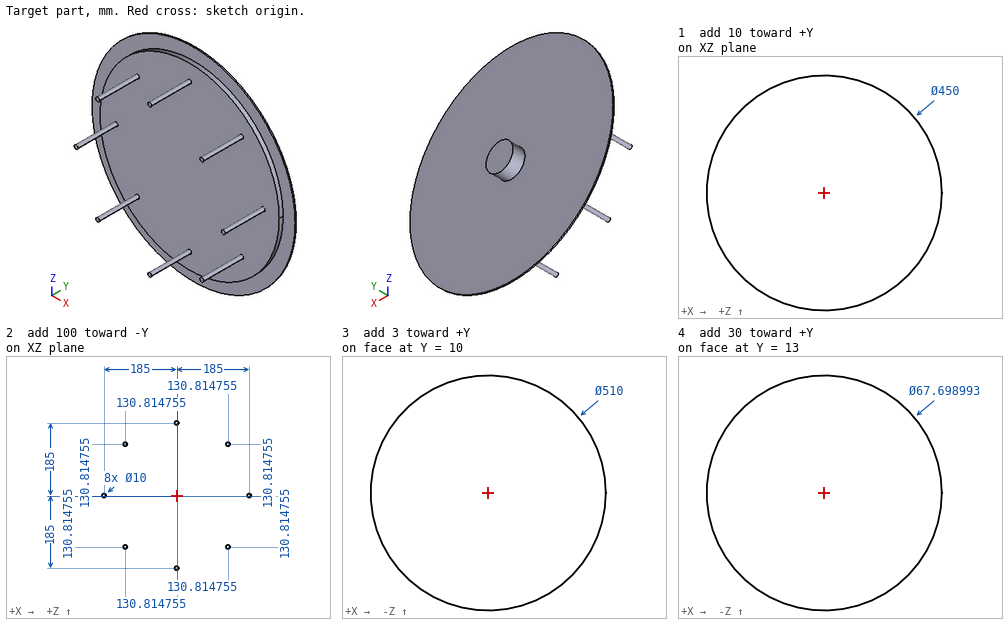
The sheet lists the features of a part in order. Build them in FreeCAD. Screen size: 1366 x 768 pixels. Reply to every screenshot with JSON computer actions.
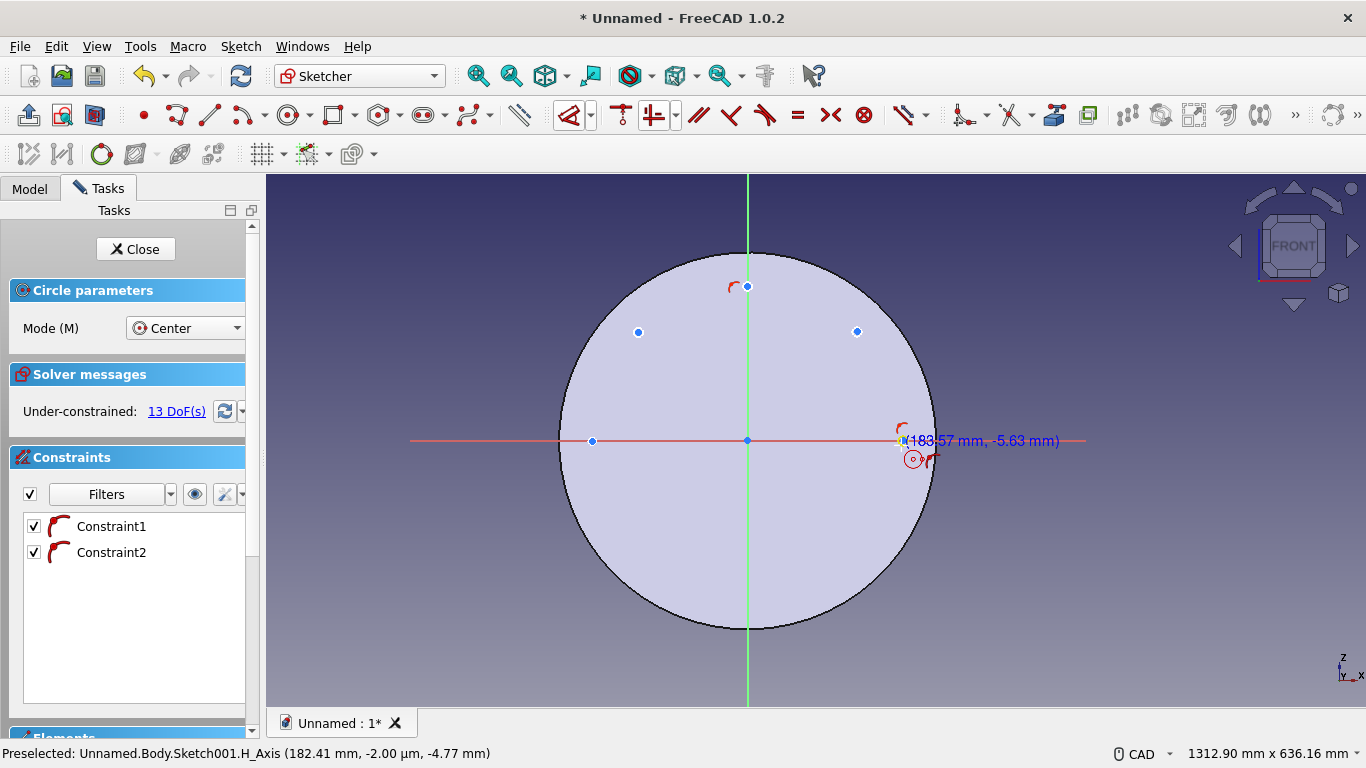
{"action": "scroll", "coordinate": [857, 551], "scroll_direction": "up", "scroll_amount": 9}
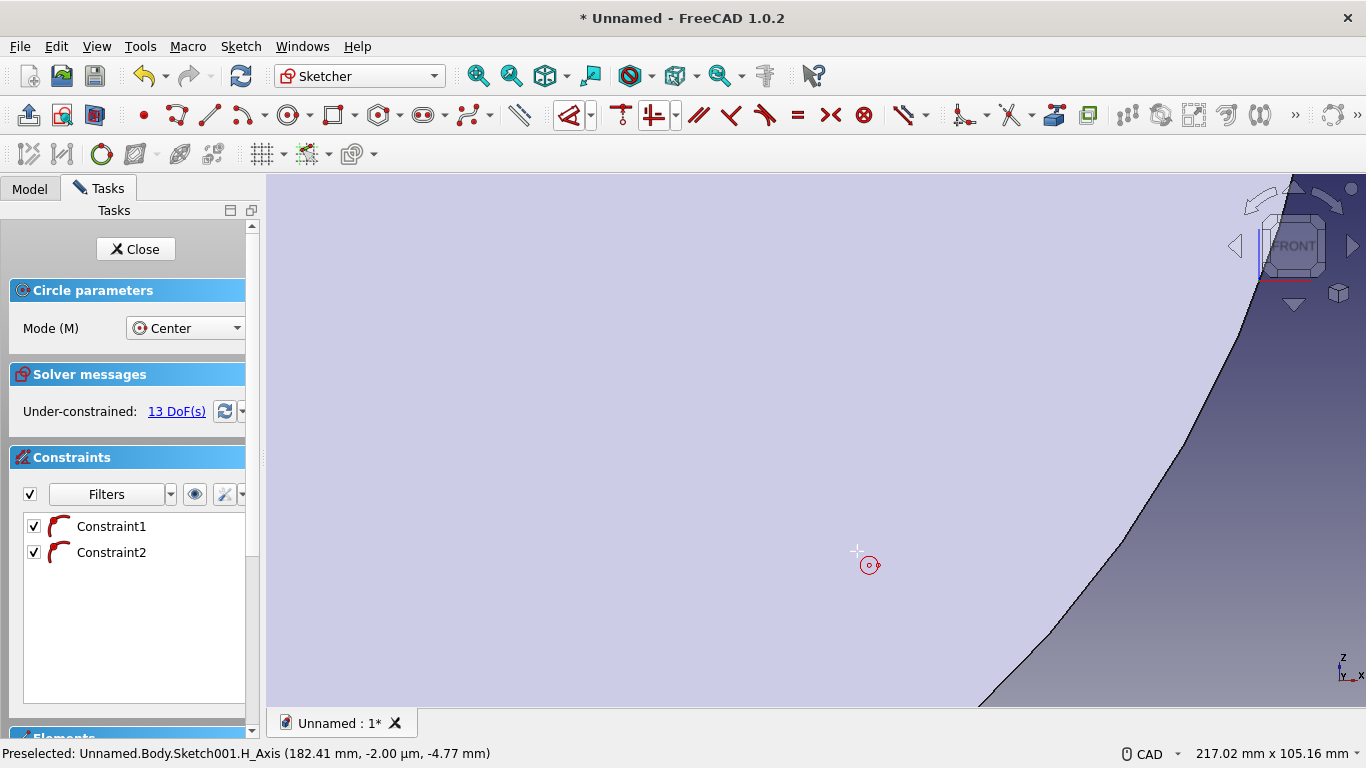
{"action": "scroll", "coordinate": [857, 551], "scroll_direction": "down", "scroll_amount": 9}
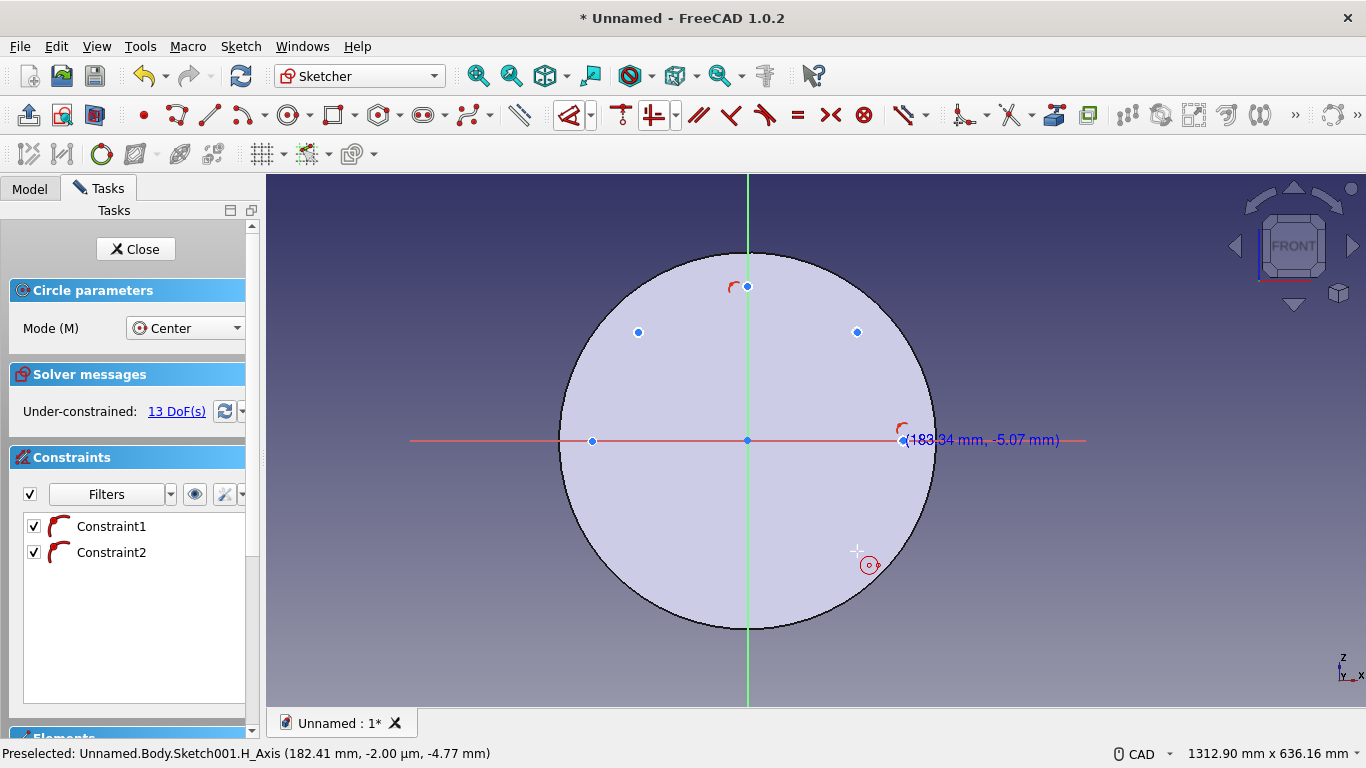
{"action": "left_click", "coordinate": [857, 551]}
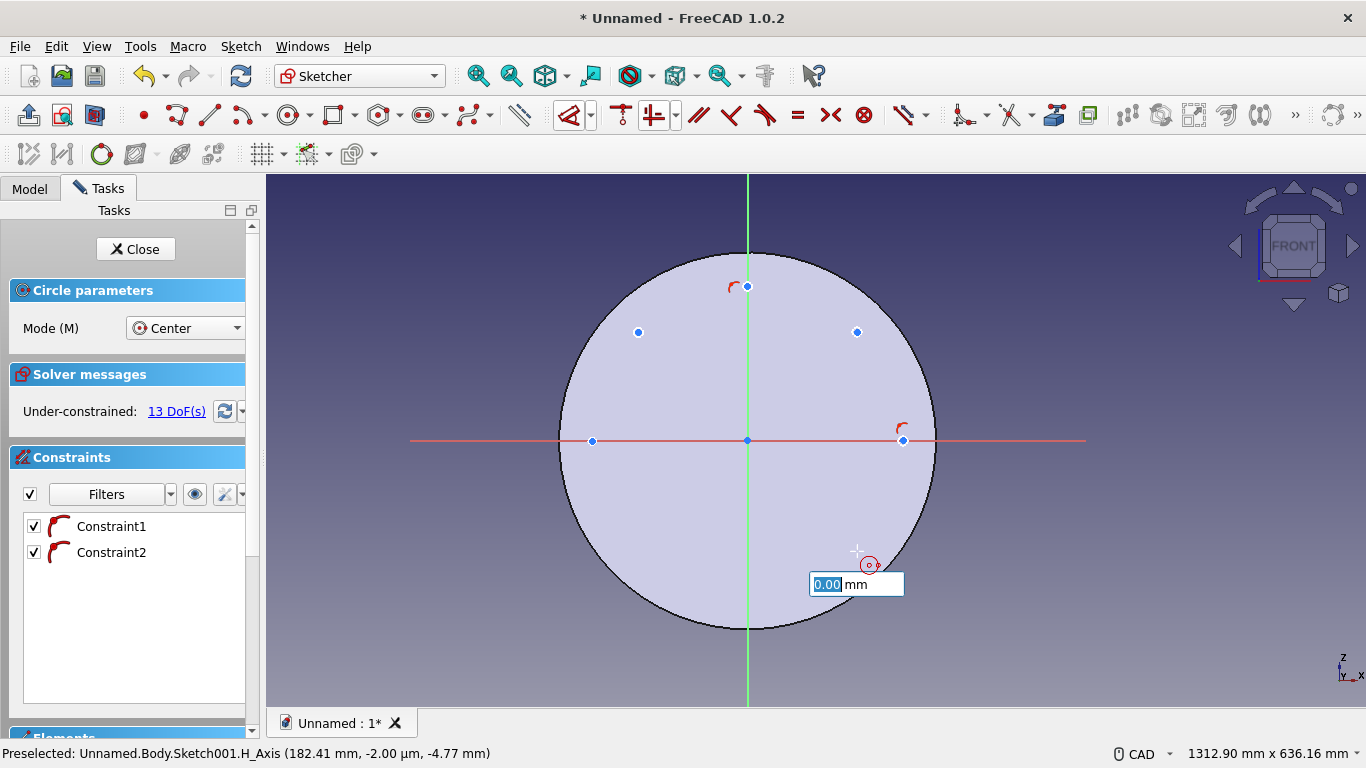
{"action": "scroll", "coordinate": [860, 548], "scroll_direction": "up", "scroll_amount": 7}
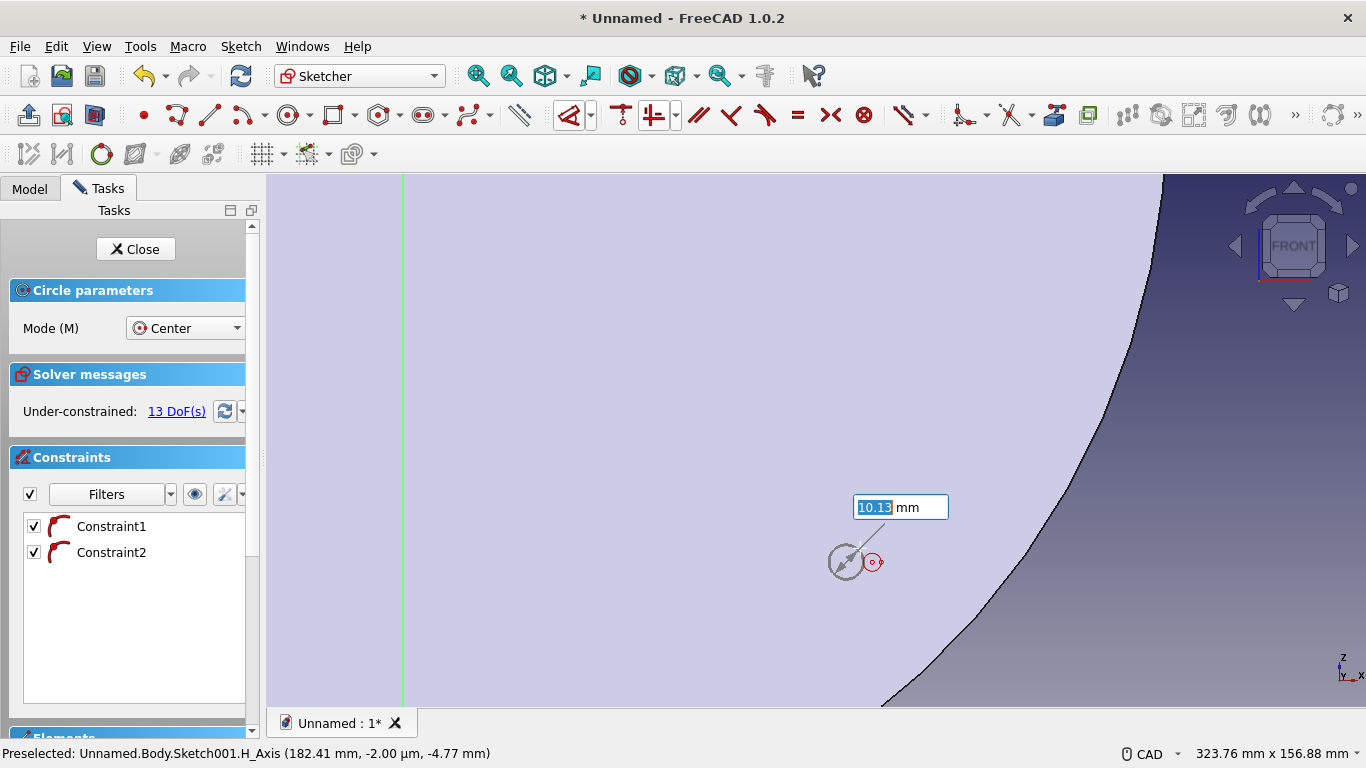
{"action": "left_click", "coordinate": [859, 544]}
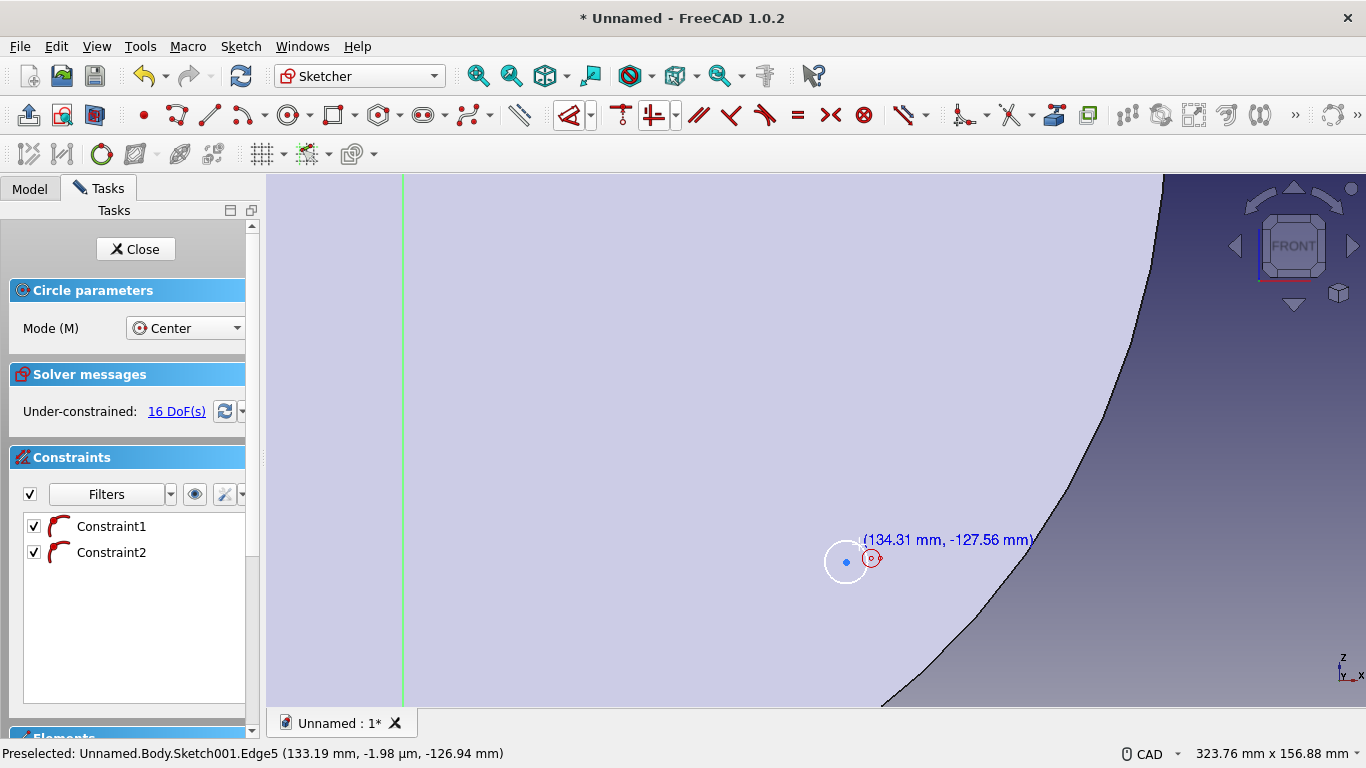
{"action": "scroll", "coordinate": [860, 548], "scroll_direction": "down", "scroll_amount": 7}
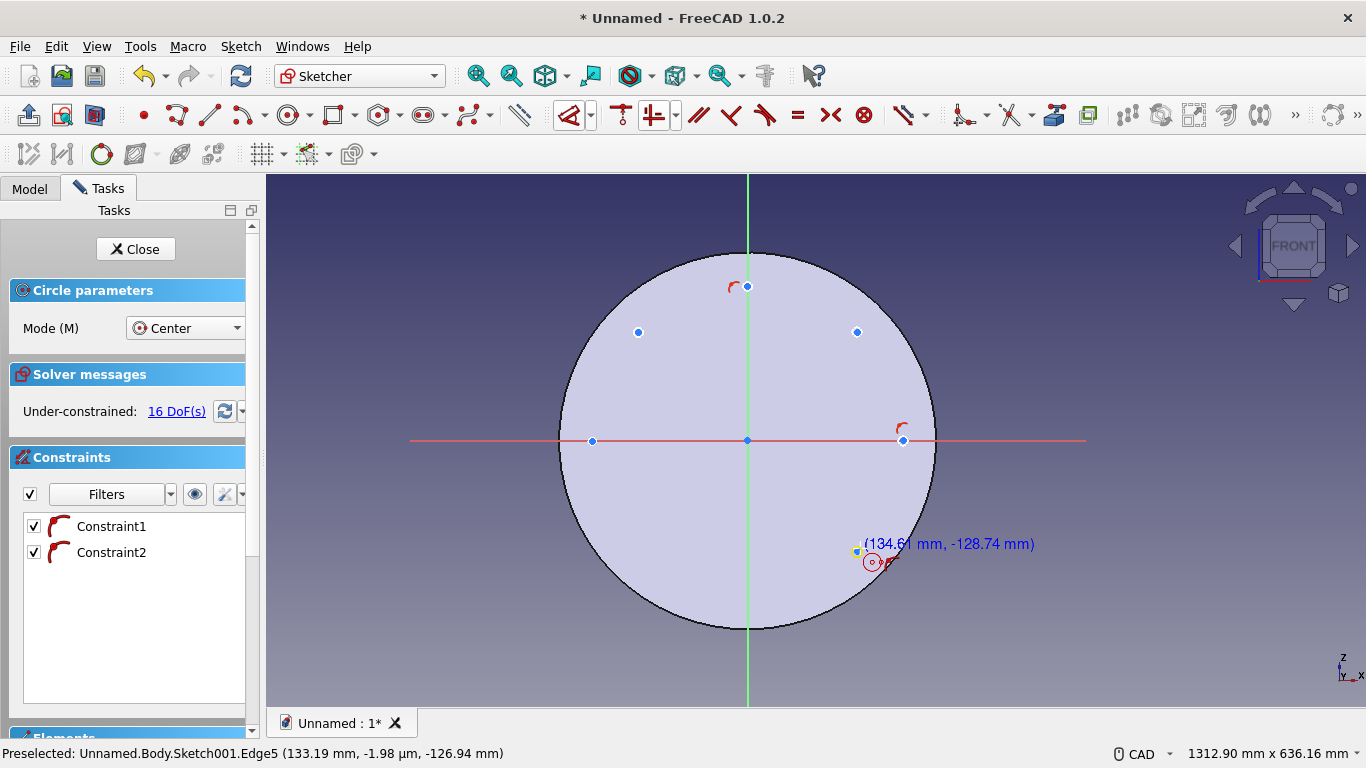
{"action": "scroll", "coordinate": [748, 596], "scroll_direction": "up", "scroll_amount": 9}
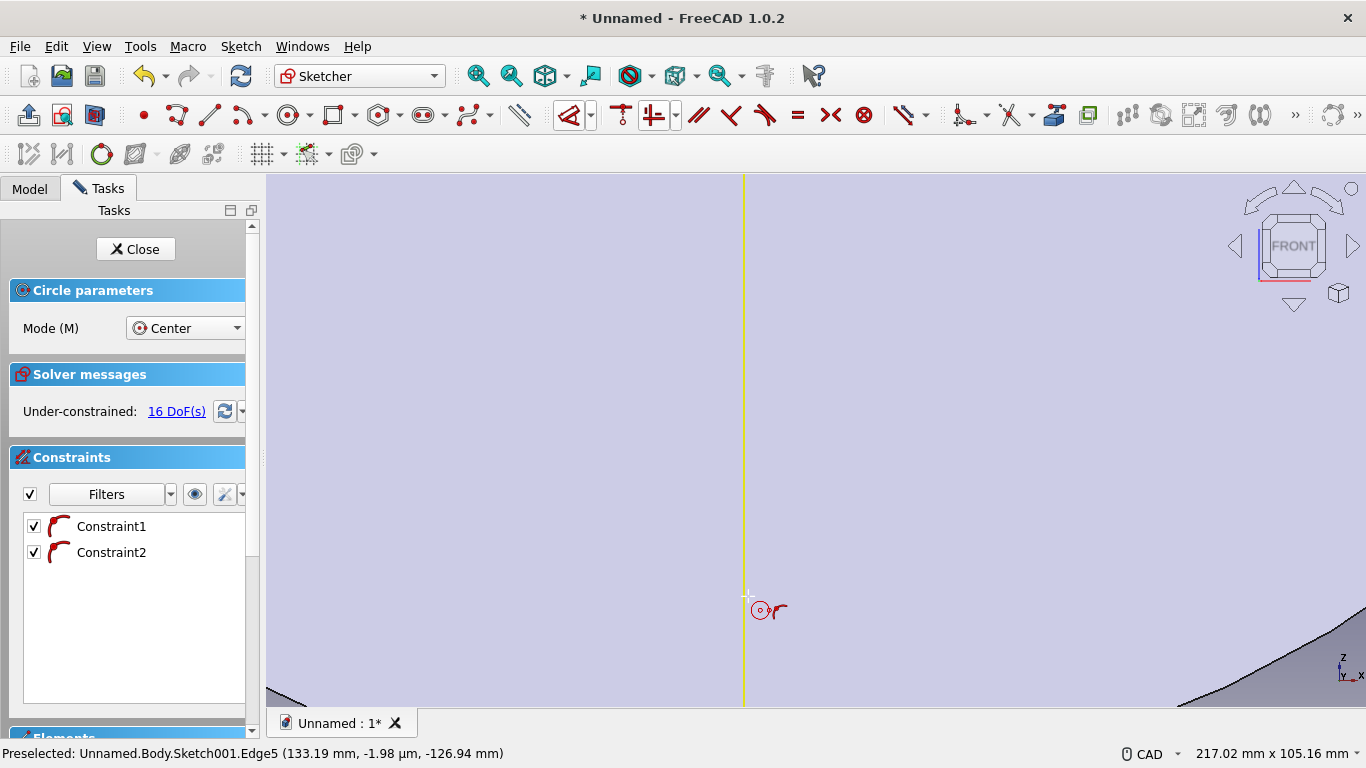
{"action": "scroll", "coordinate": [748, 596], "scroll_direction": "down", "scroll_amount": 9}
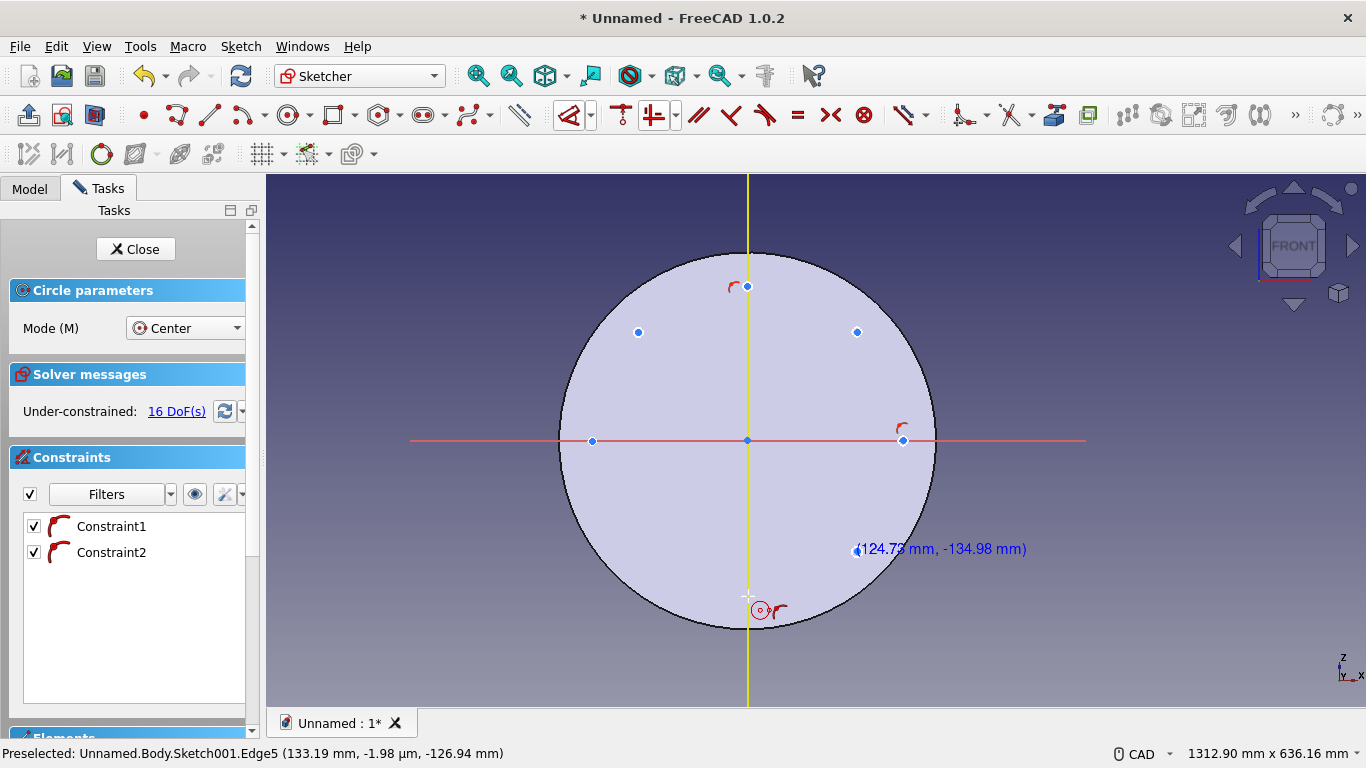
{"action": "left_click", "coordinate": [748, 596]}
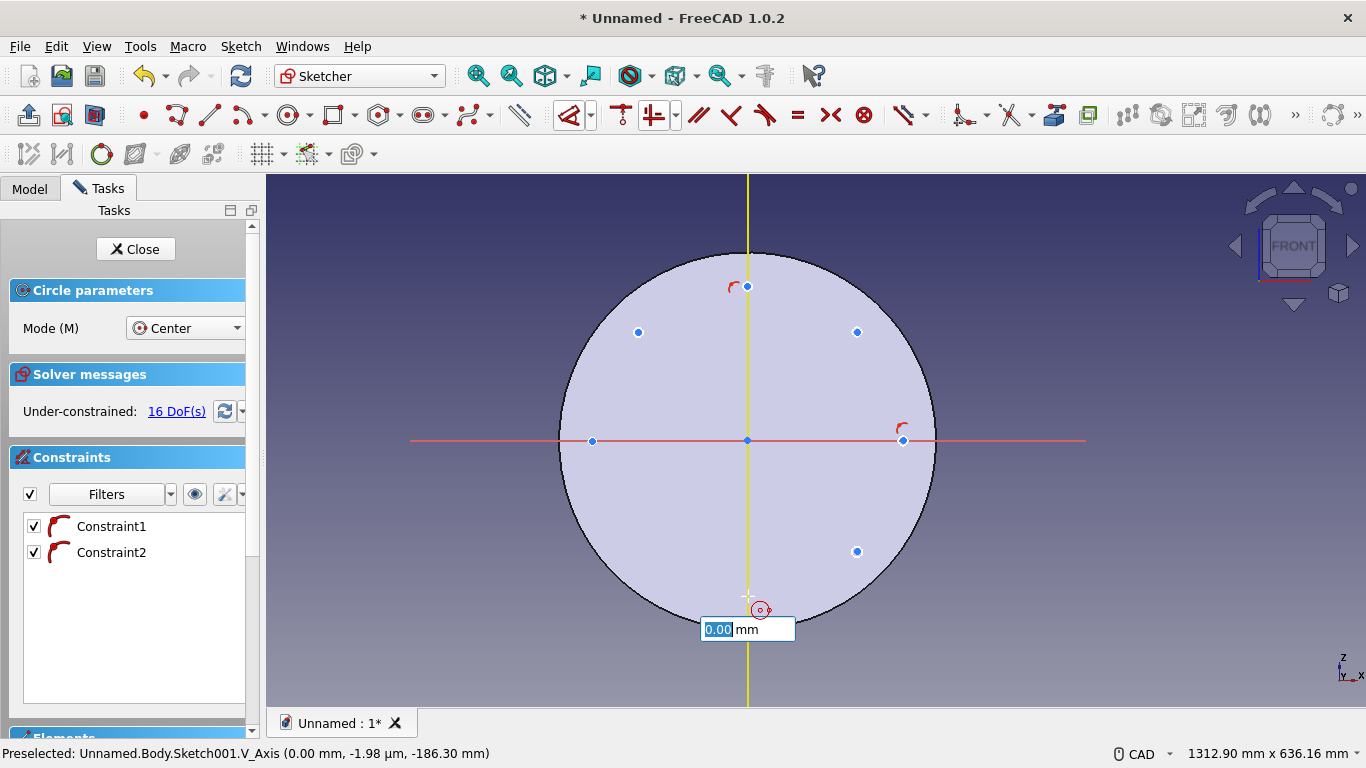
{"action": "scroll", "coordinate": [752, 594], "scroll_direction": "up", "scroll_amount": 7}